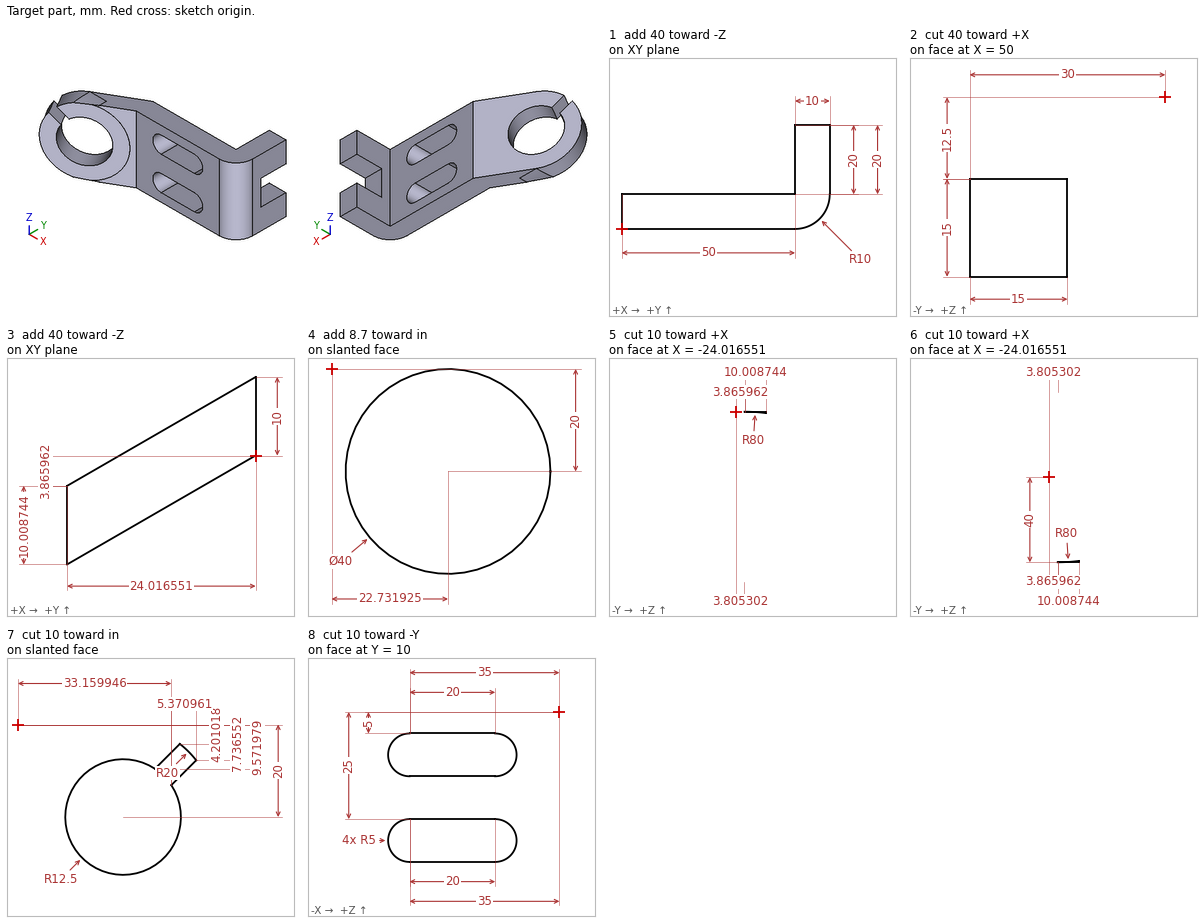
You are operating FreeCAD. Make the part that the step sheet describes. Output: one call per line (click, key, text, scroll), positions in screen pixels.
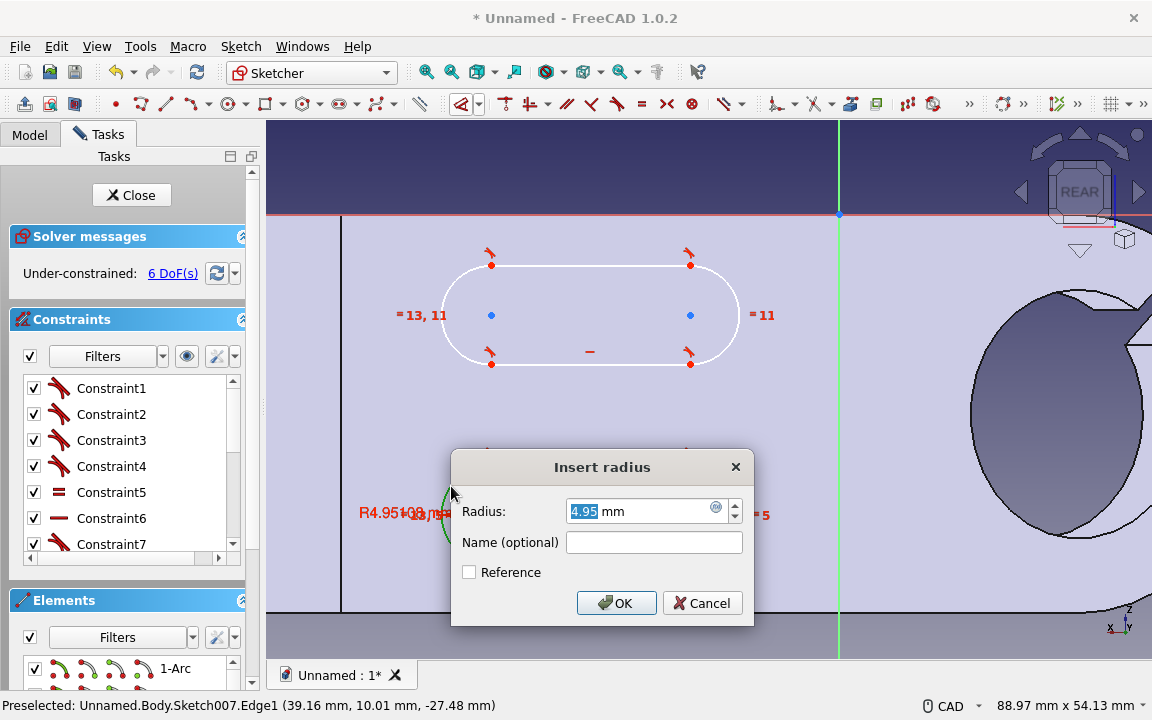
text(5)
key(Return)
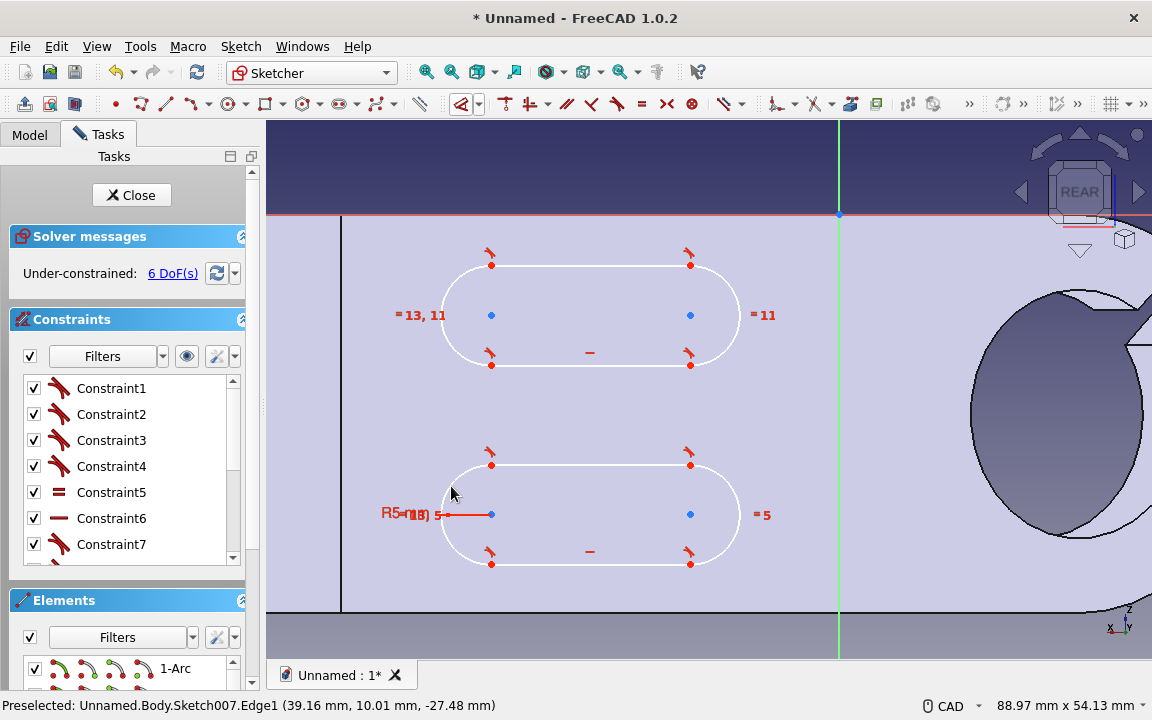
click(551, 465)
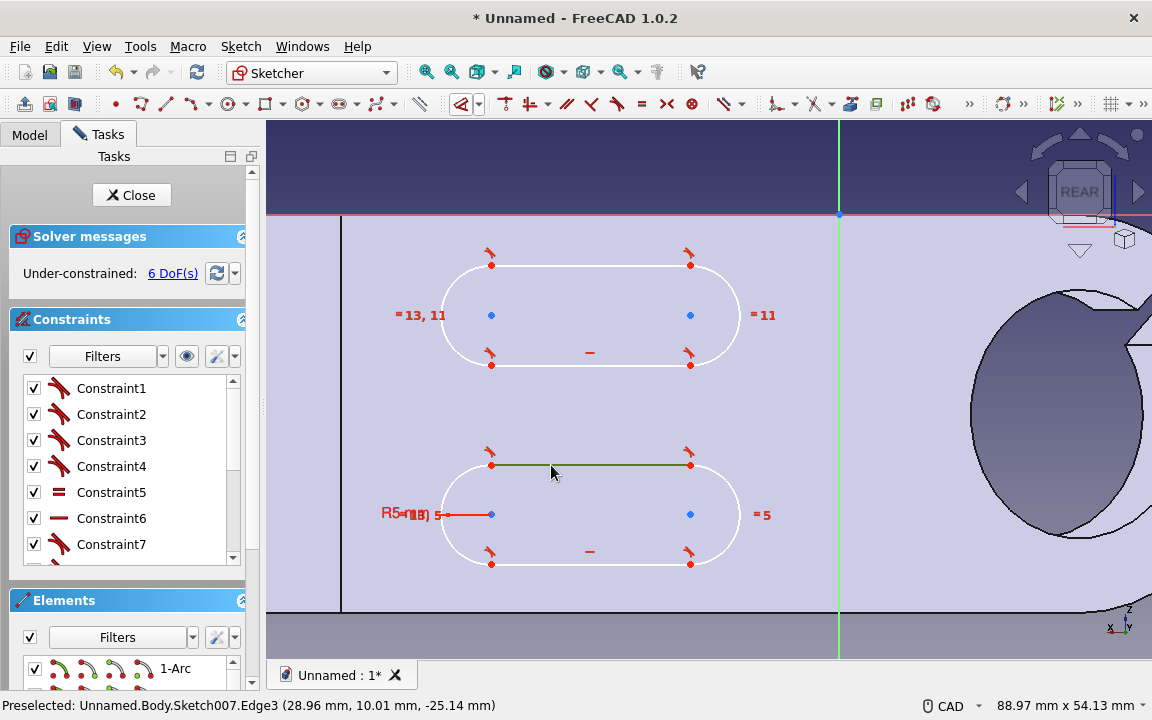
key(l)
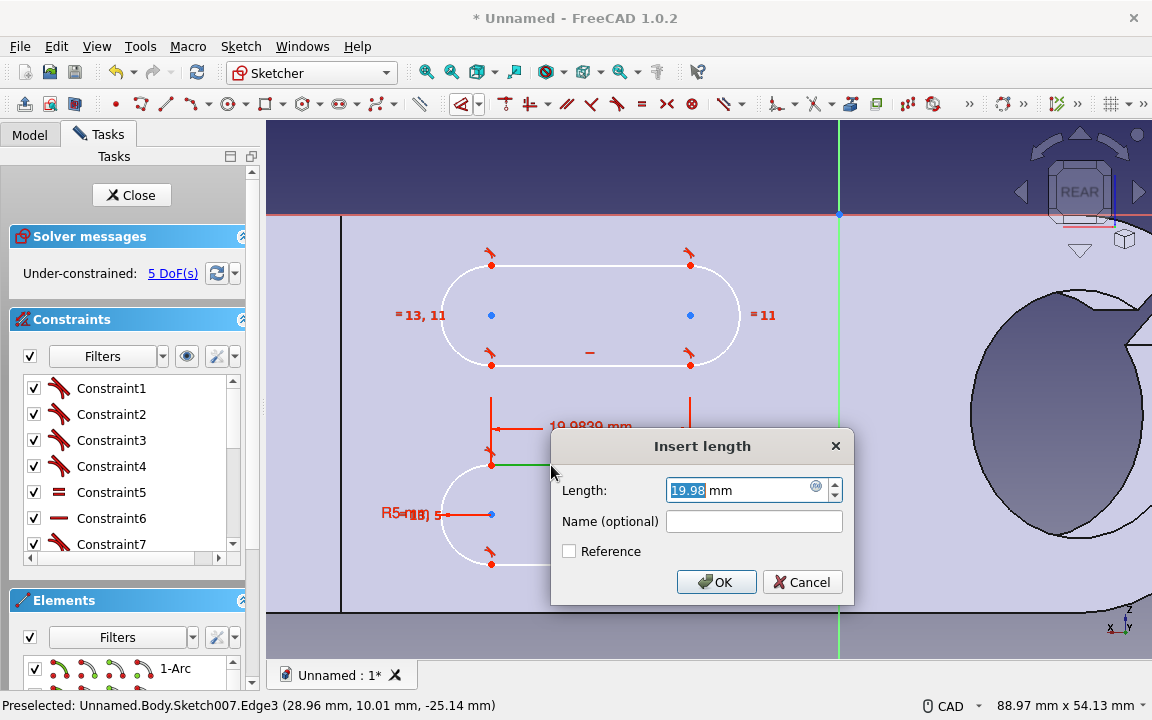
text(20)
key(Return)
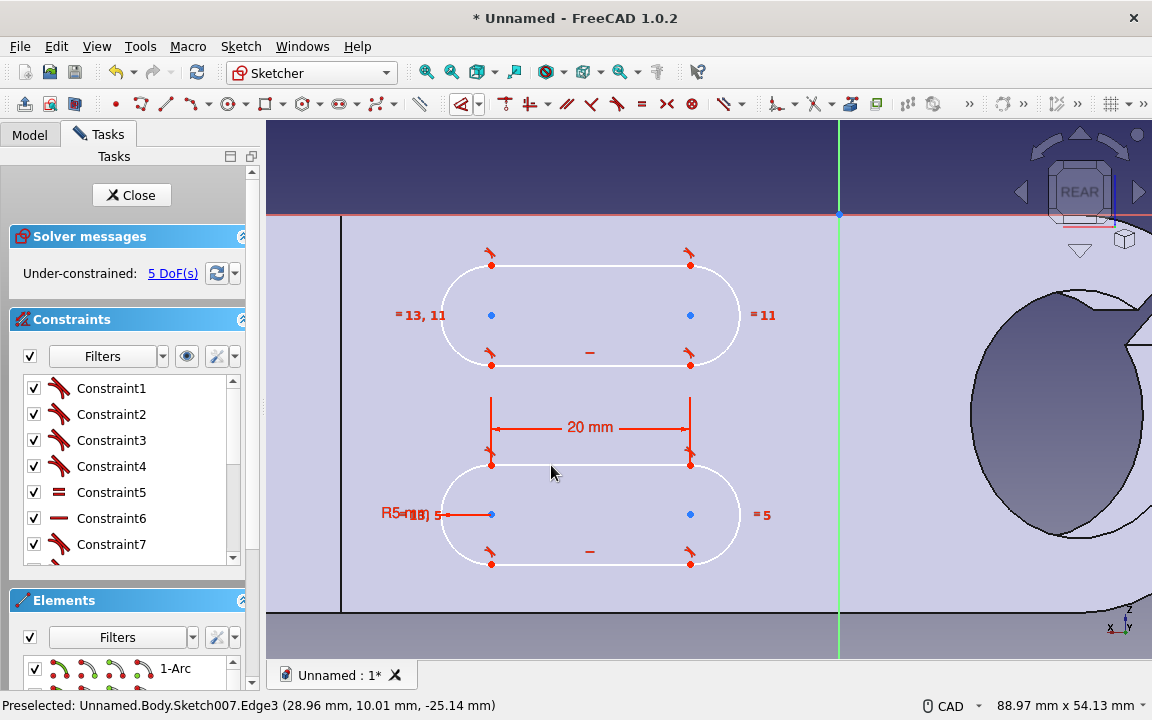
click(551, 266)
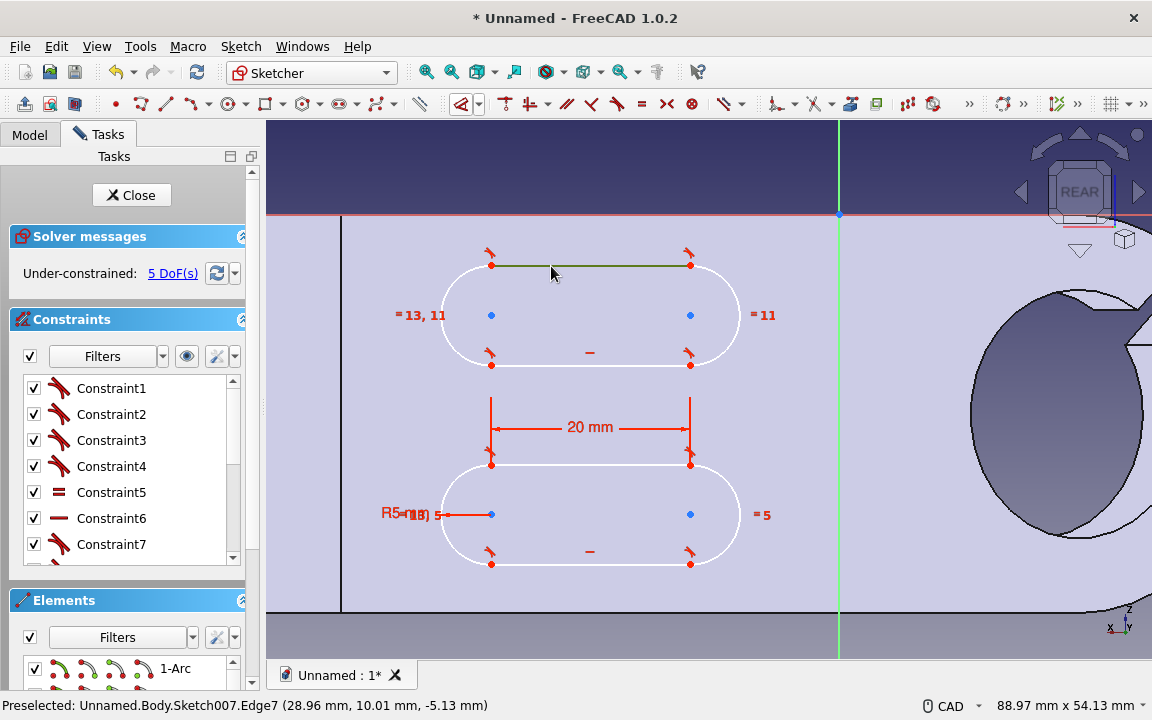
key(l)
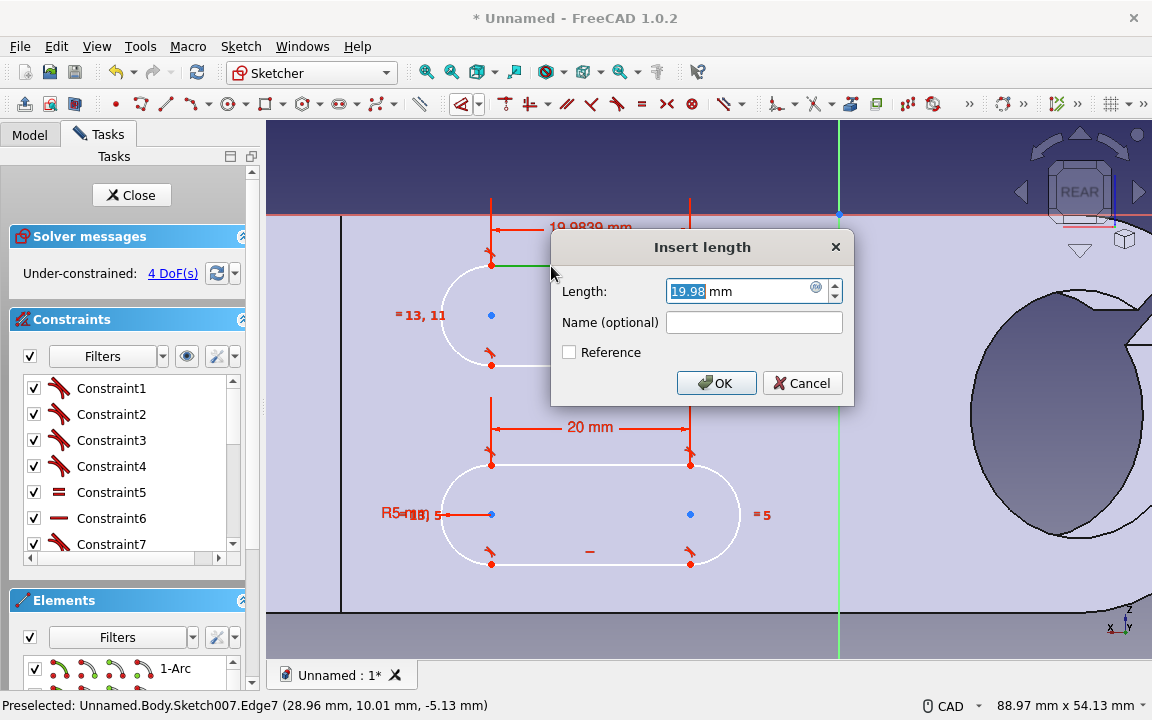
text(20)
key(Return)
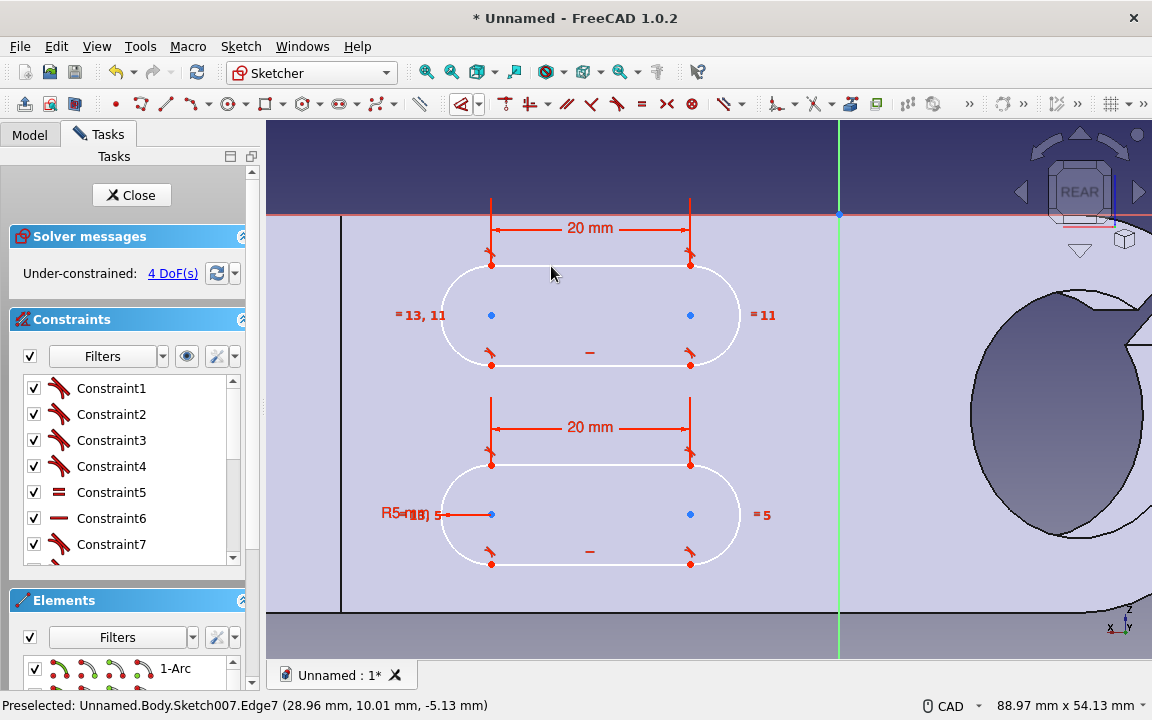
click(491, 266)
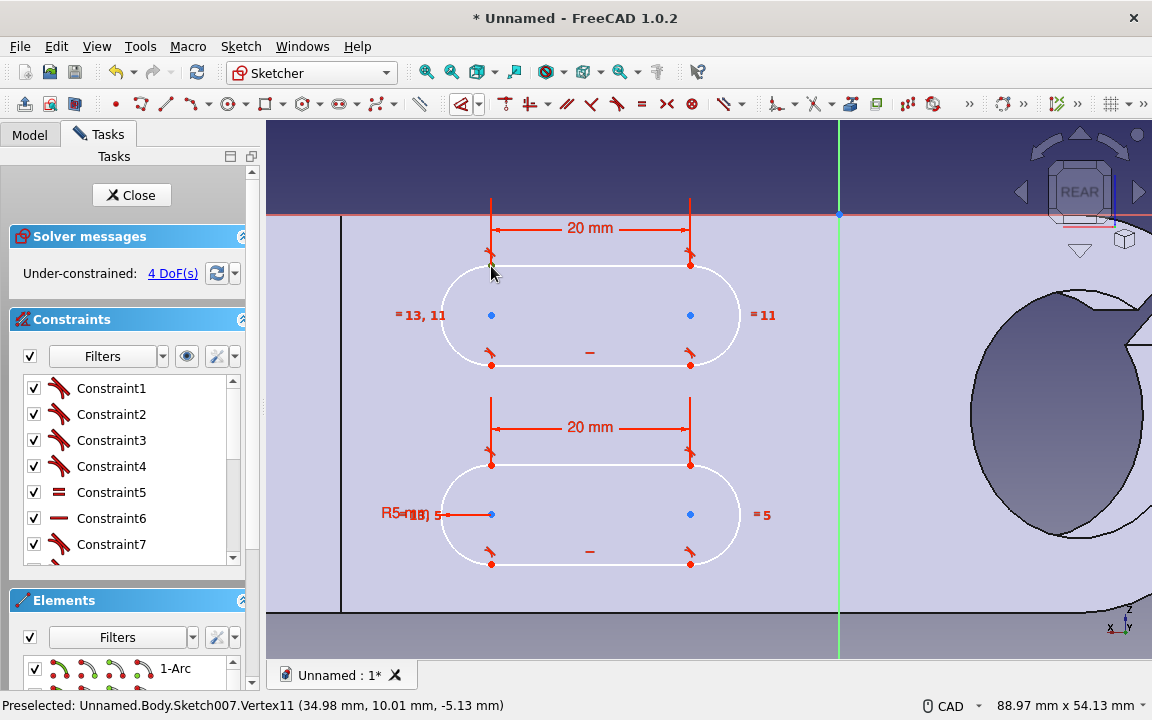
click(478, 104)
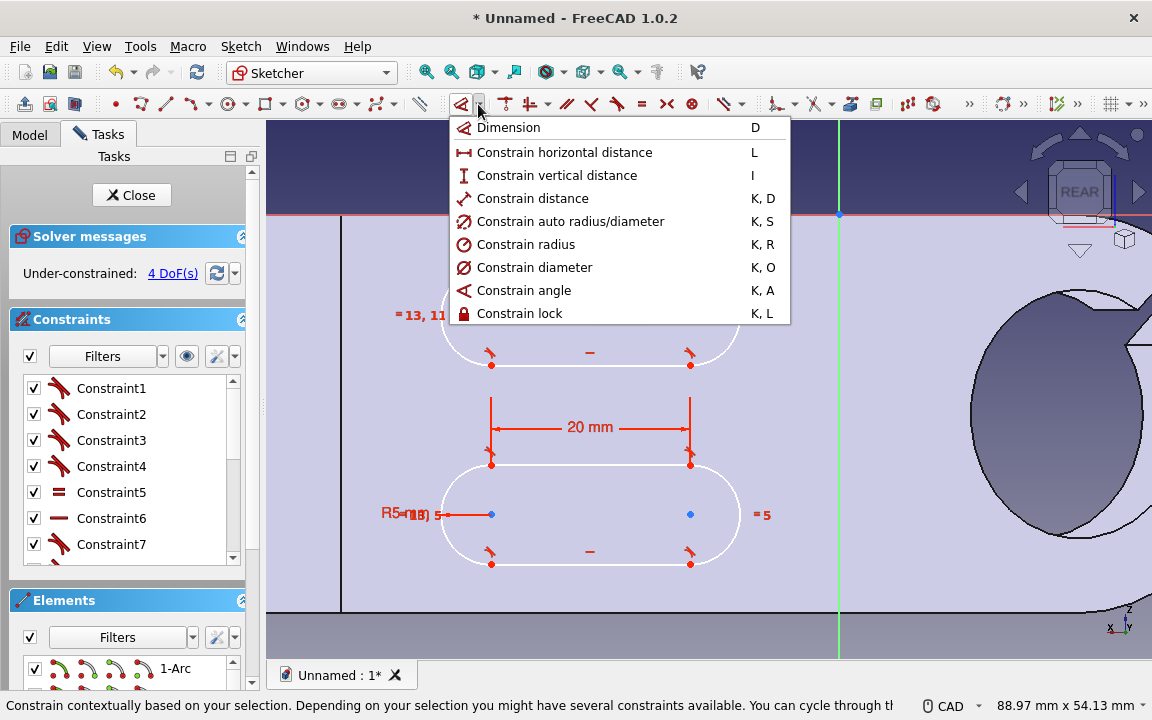
click(620, 176)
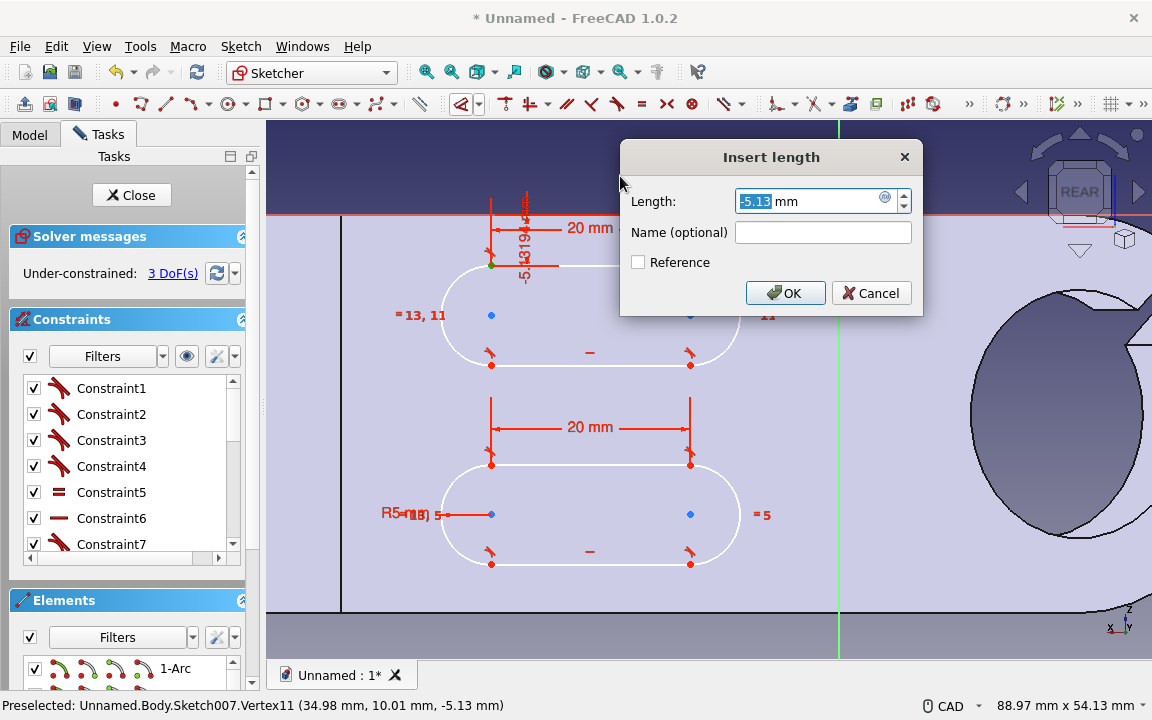
text(-5)
key(Return)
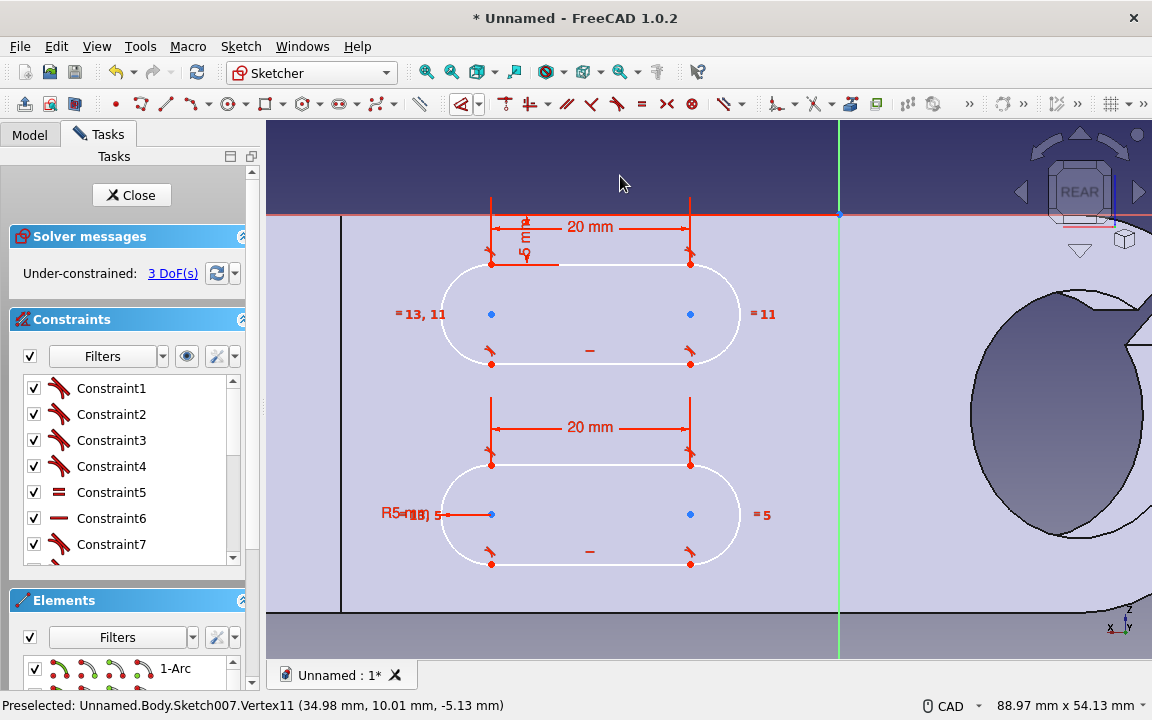
click(491, 465)